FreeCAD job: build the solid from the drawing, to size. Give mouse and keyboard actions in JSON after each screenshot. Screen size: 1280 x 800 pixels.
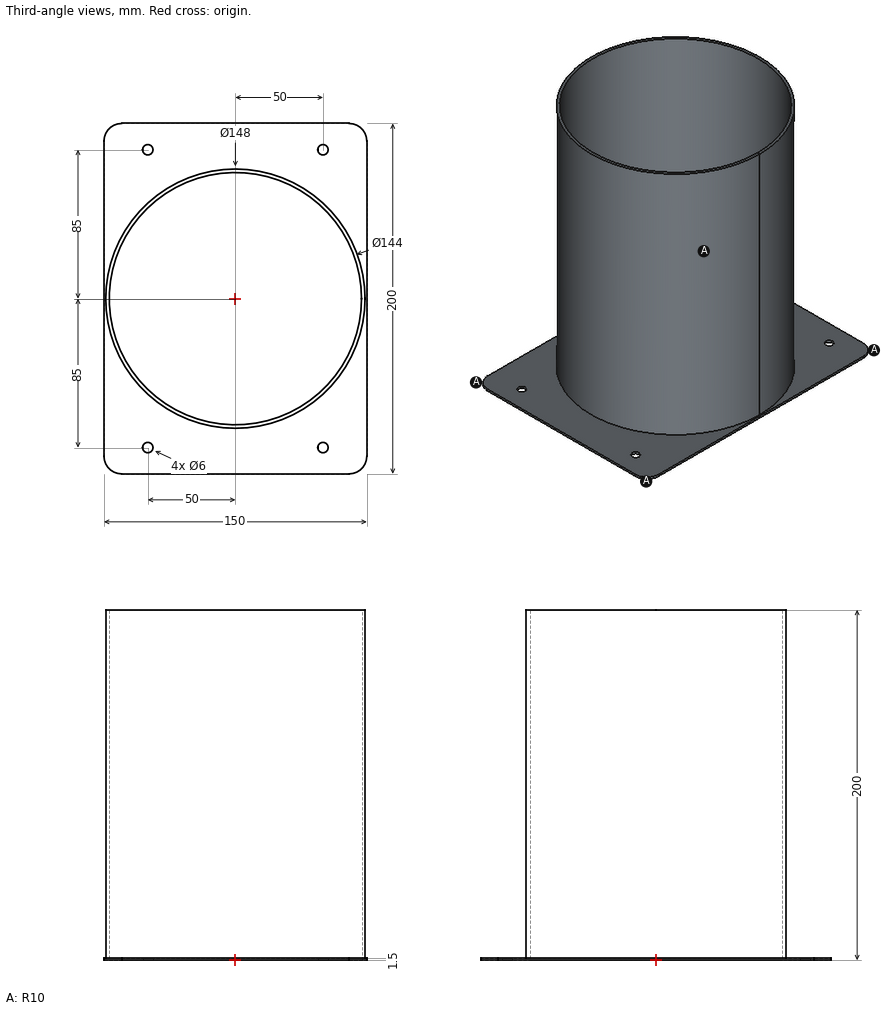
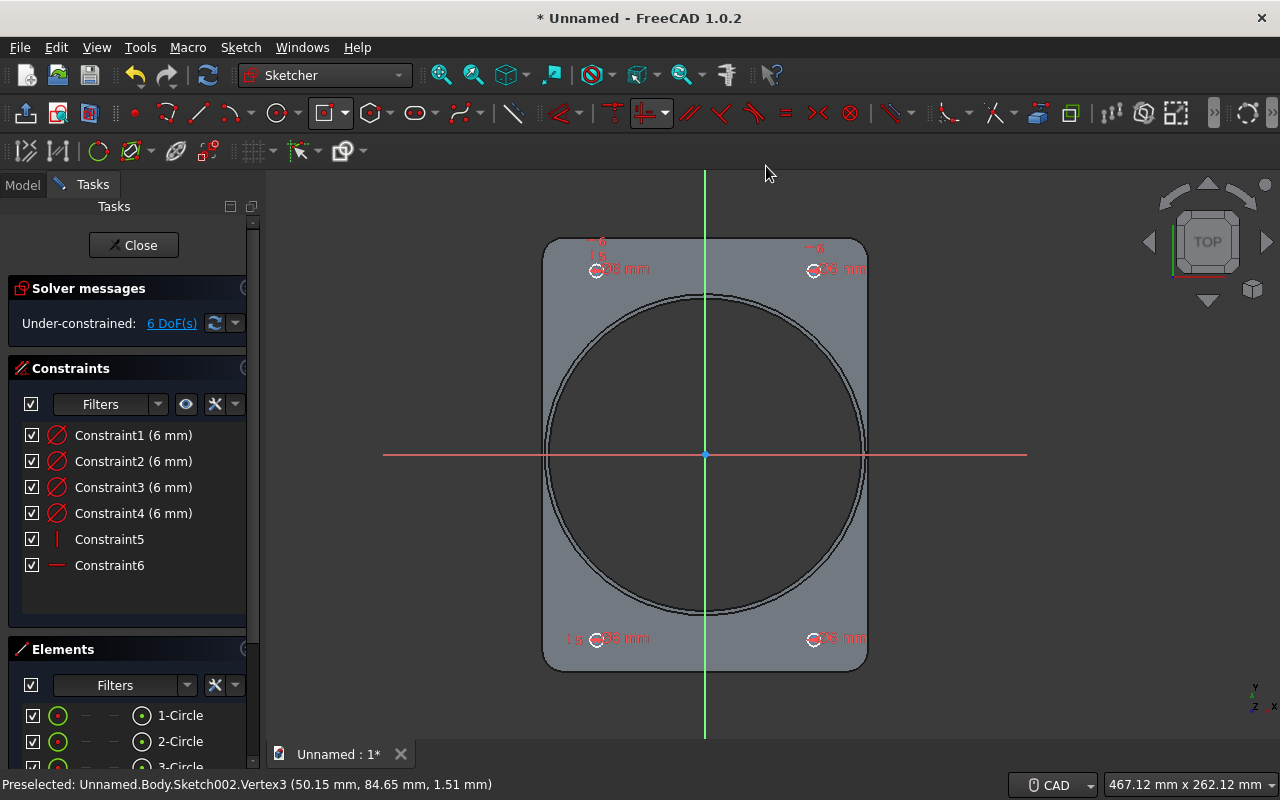
{"action": "left_click", "coordinate": [814, 271]}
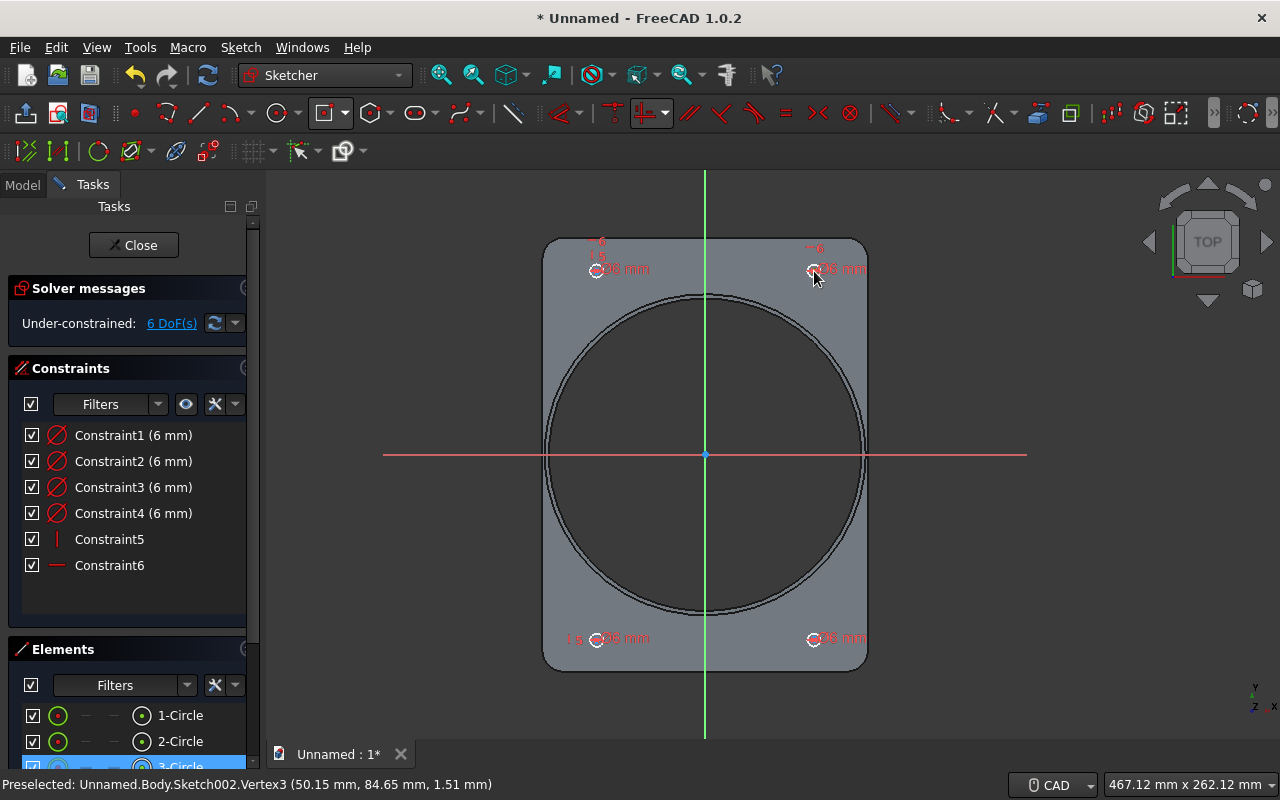
{"action": "left_click", "coordinate": [814, 640]}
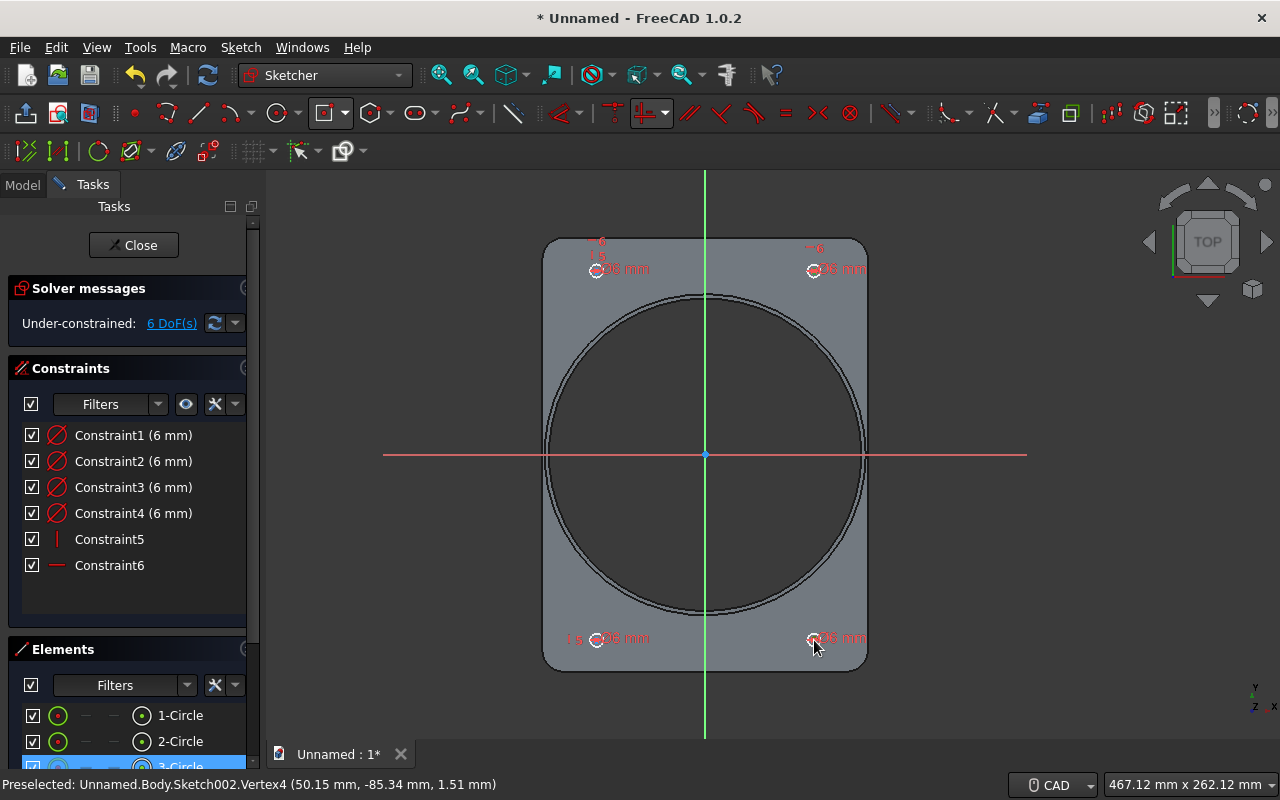
{"action": "key", "text": "v"}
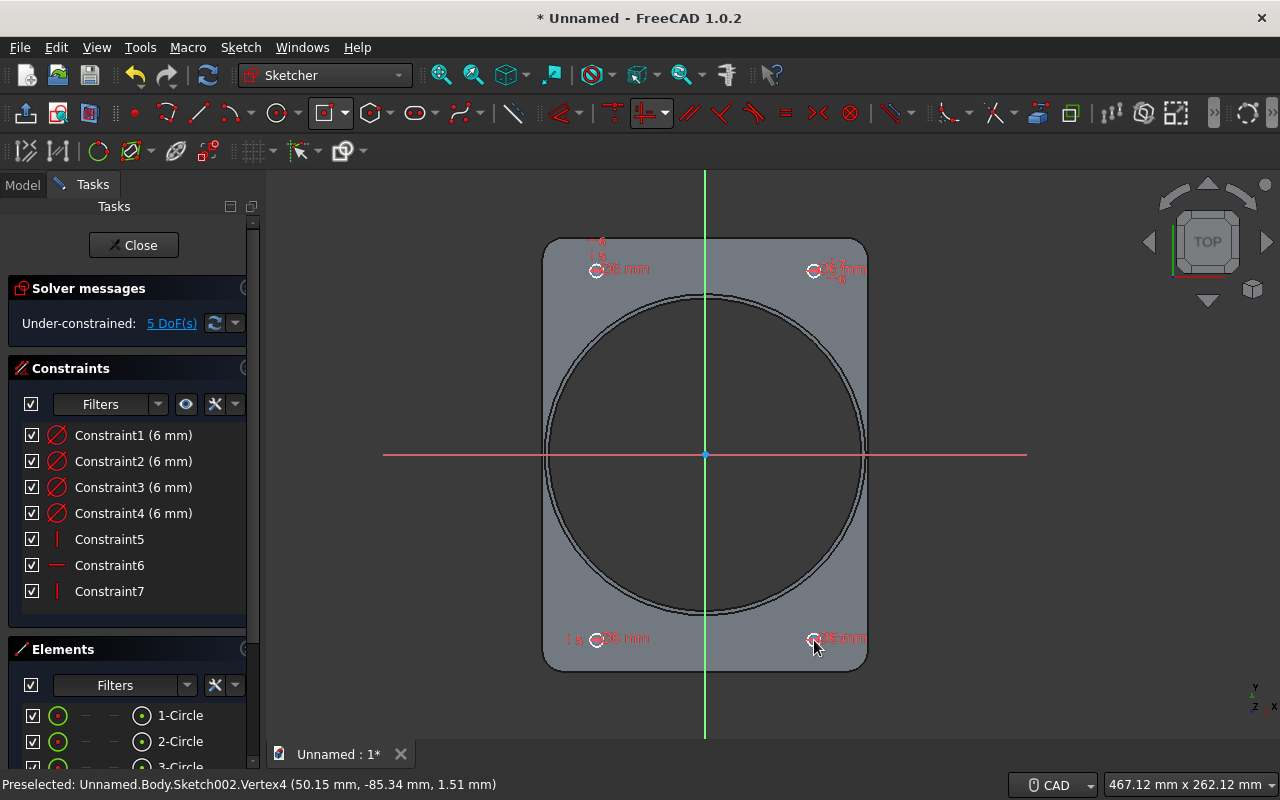
{"action": "left_click", "coordinate": [597, 640]}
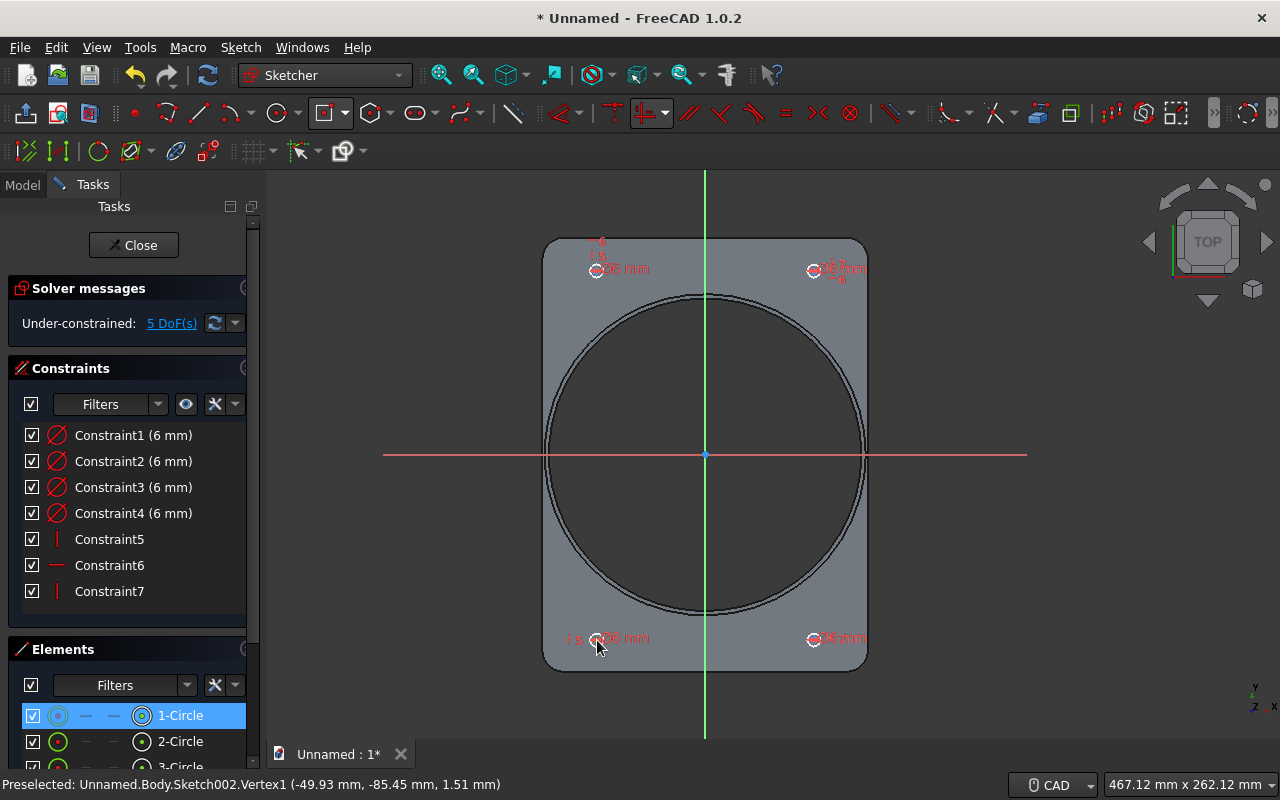
{"action": "left_click", "coordinate": [814, 640]}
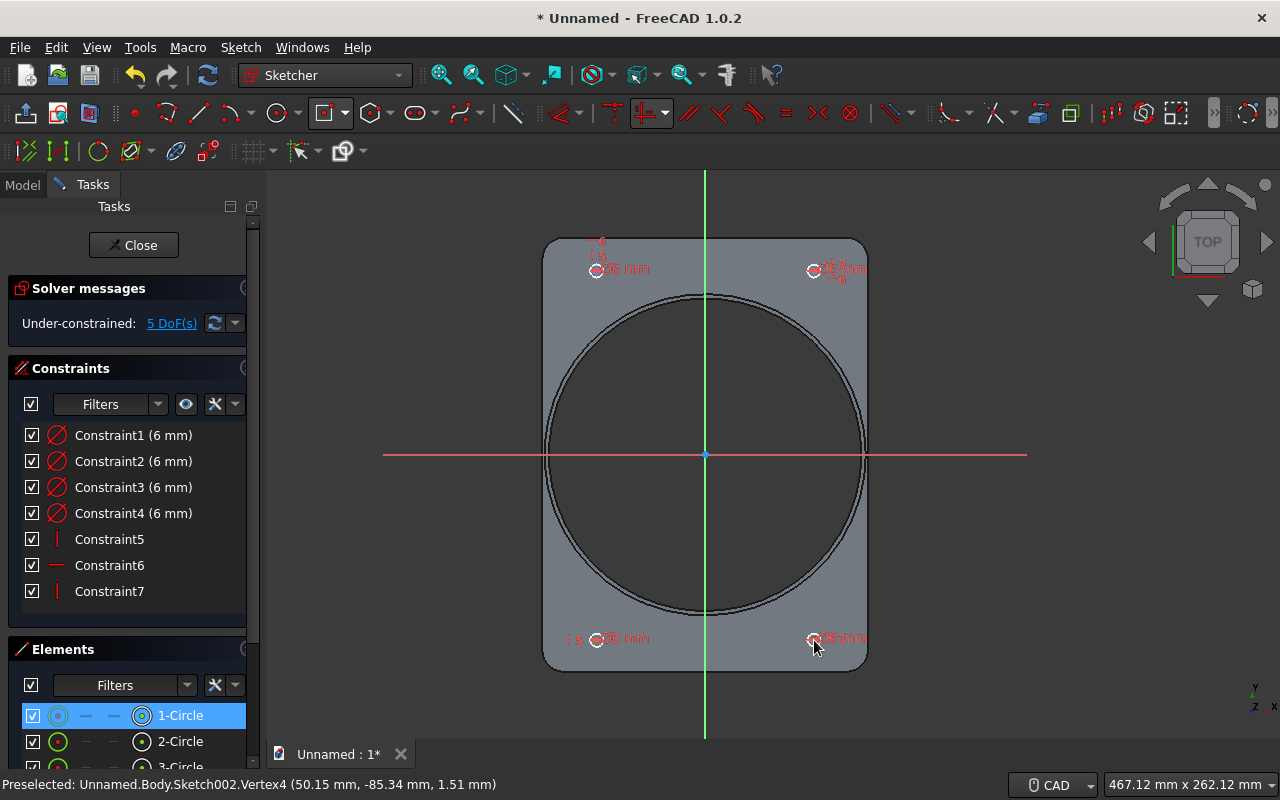
{"action": "key", "text": "h"}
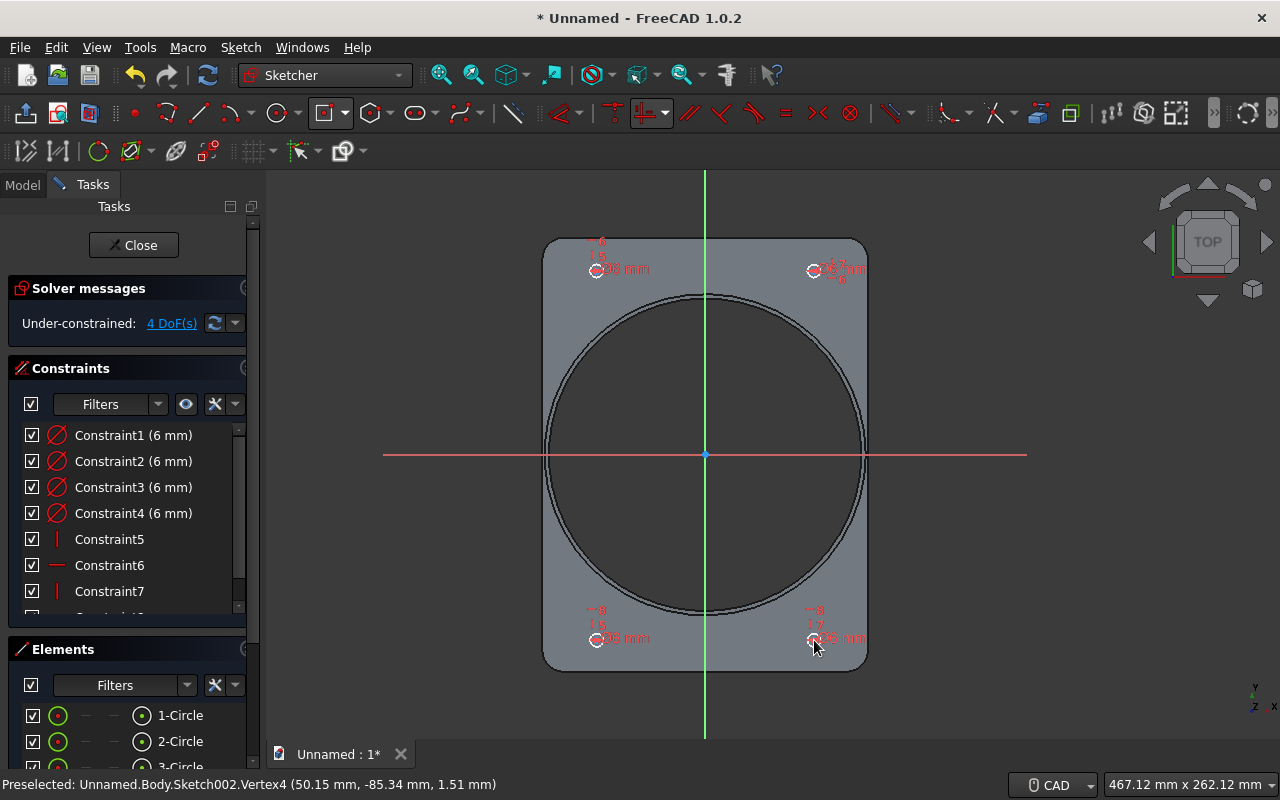
{"action": "left_click", "coordinate": [560, 114]}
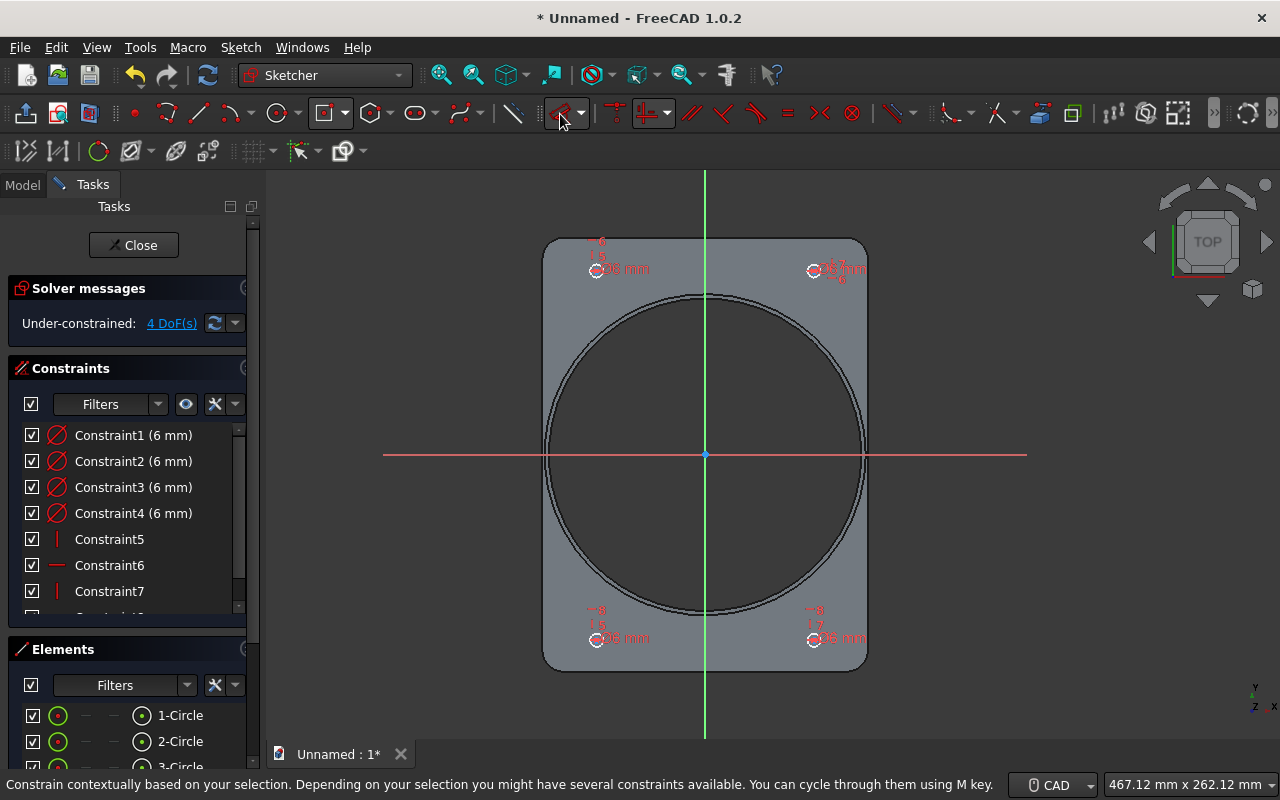
{"action": "left_click", "coordinate": [597, 640]}
{"action": "left_click", "coordinate": [651, 674]}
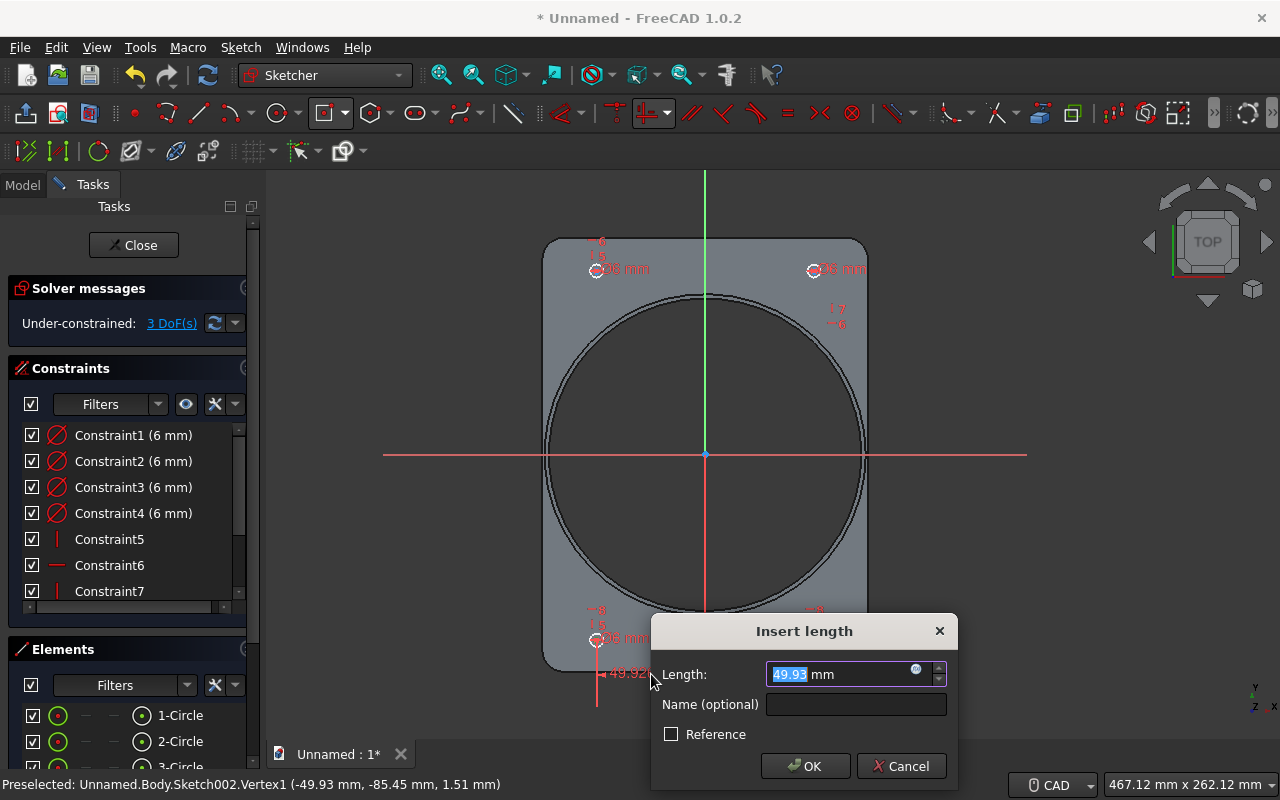
{"action": "type", "text": "50"}
{"action": "key", "text": "Return"}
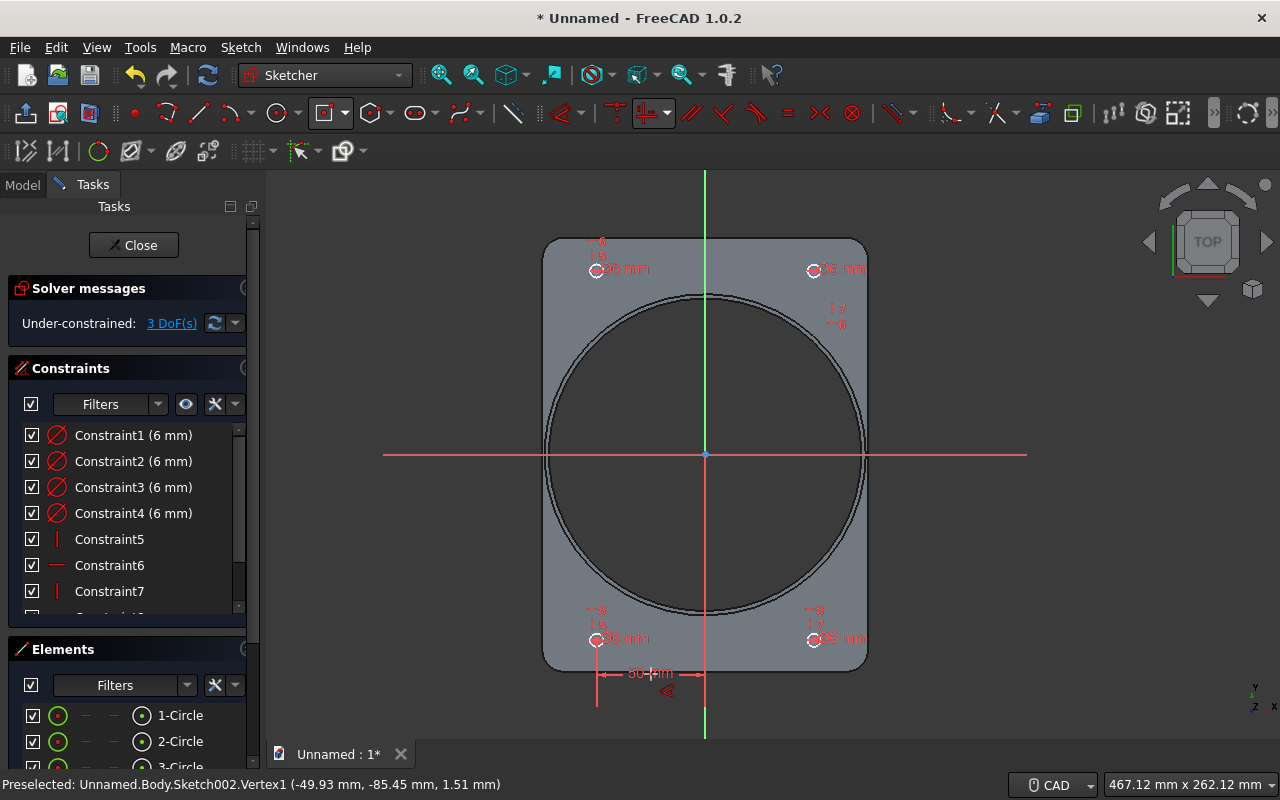
{"action": "left_click", "coordinate": [597, 640]}
{"action": "left_click", "coordinate": [563, 547]}